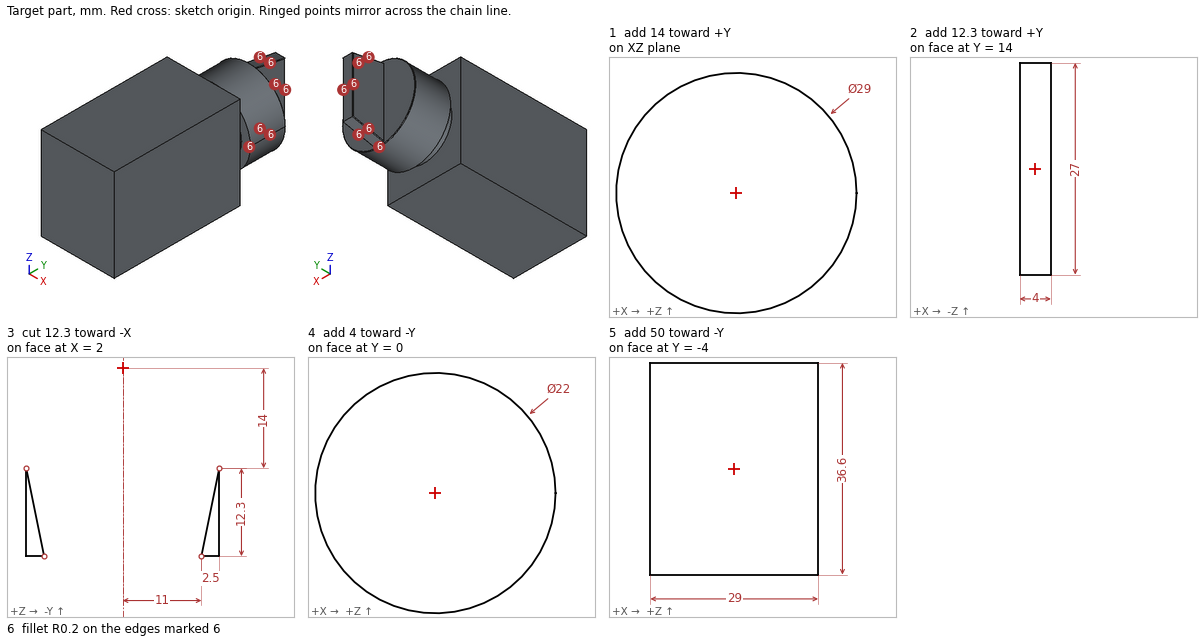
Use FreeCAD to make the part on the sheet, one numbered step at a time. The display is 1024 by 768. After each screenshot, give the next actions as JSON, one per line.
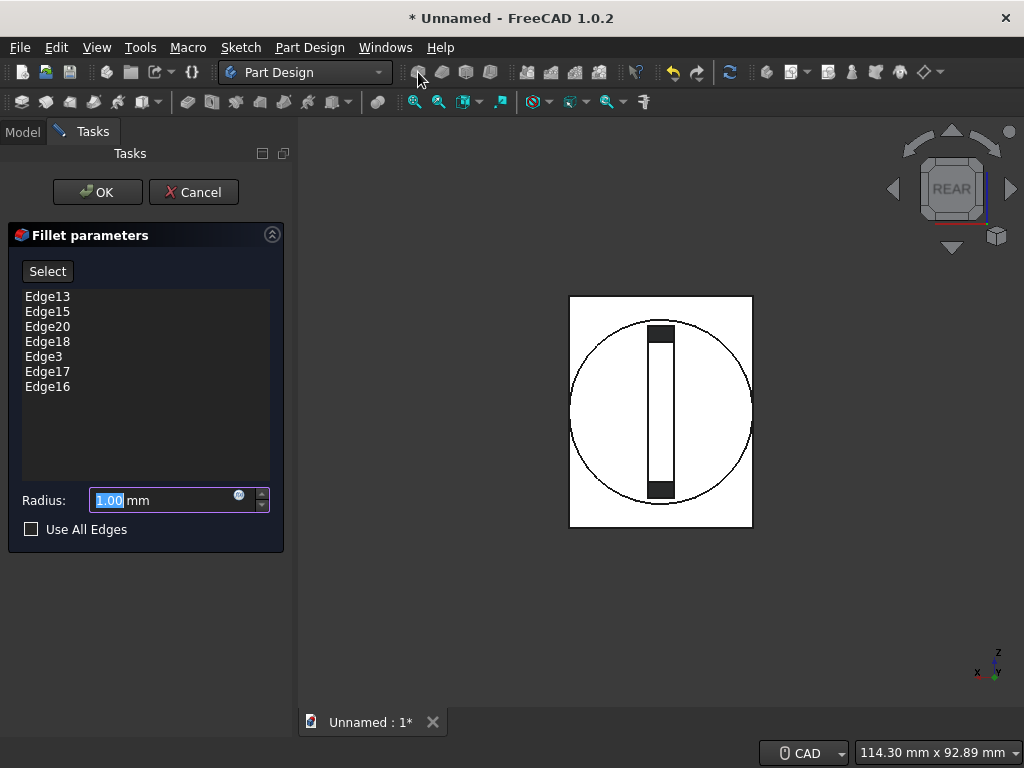
{"action": "type", "text": "0.2"}
{"action": "key", "text": "Tab"}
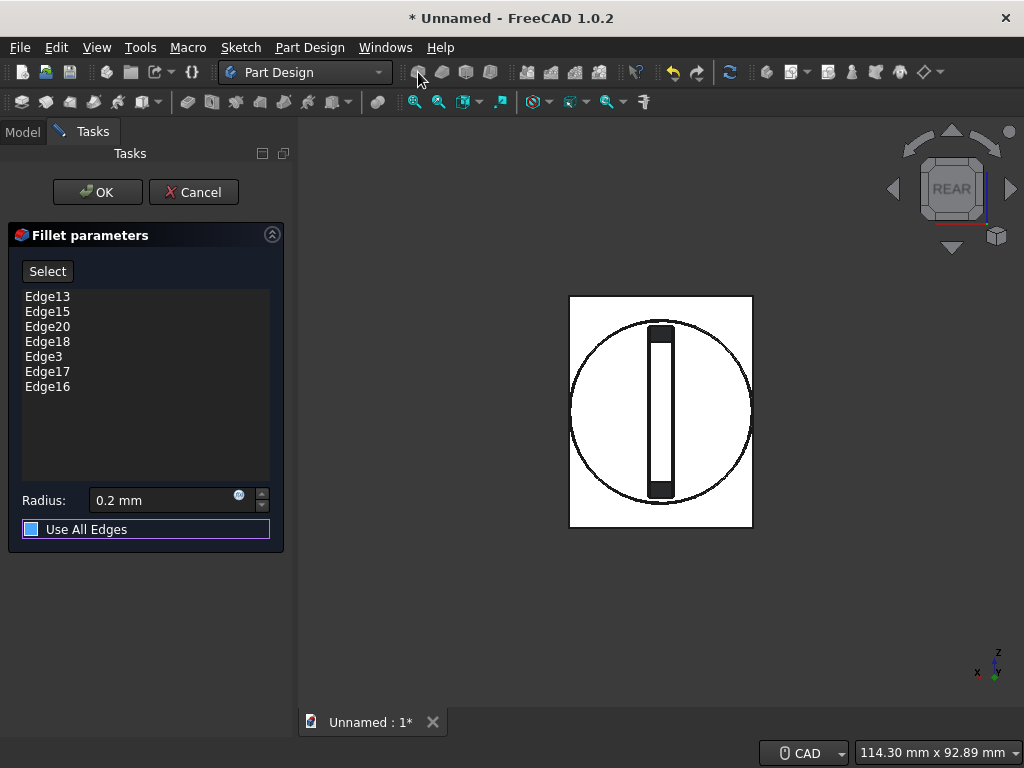
{"action": "left_click", "coordinate": [98, 192]}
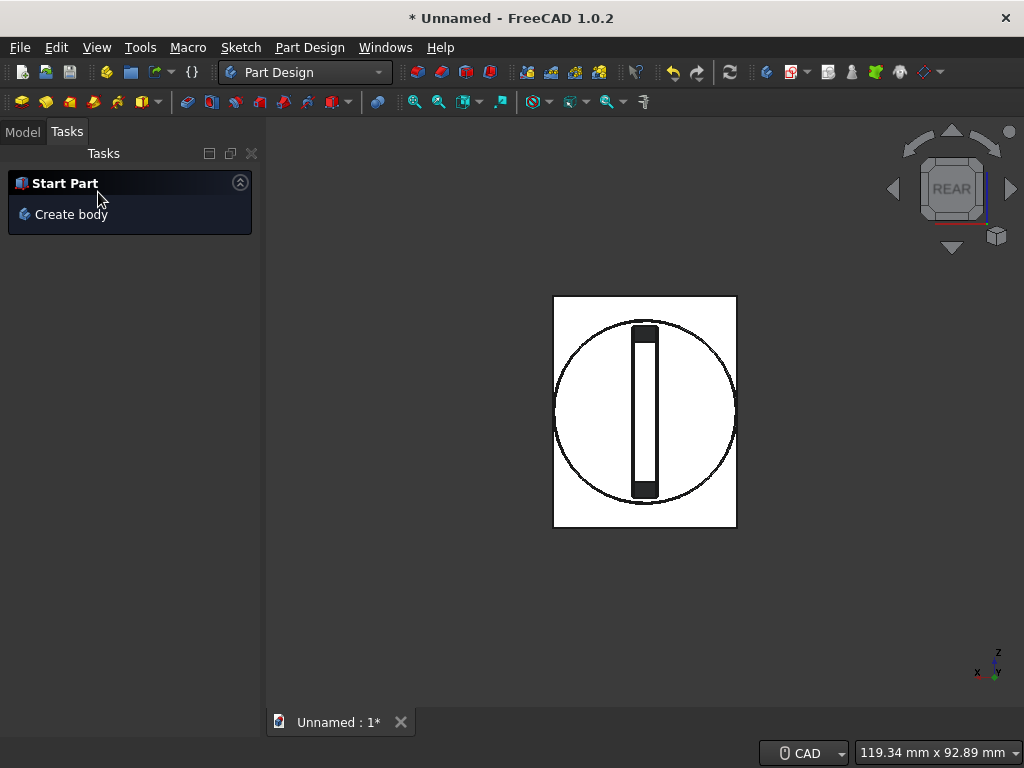
{"action": "key", "text": "0"}